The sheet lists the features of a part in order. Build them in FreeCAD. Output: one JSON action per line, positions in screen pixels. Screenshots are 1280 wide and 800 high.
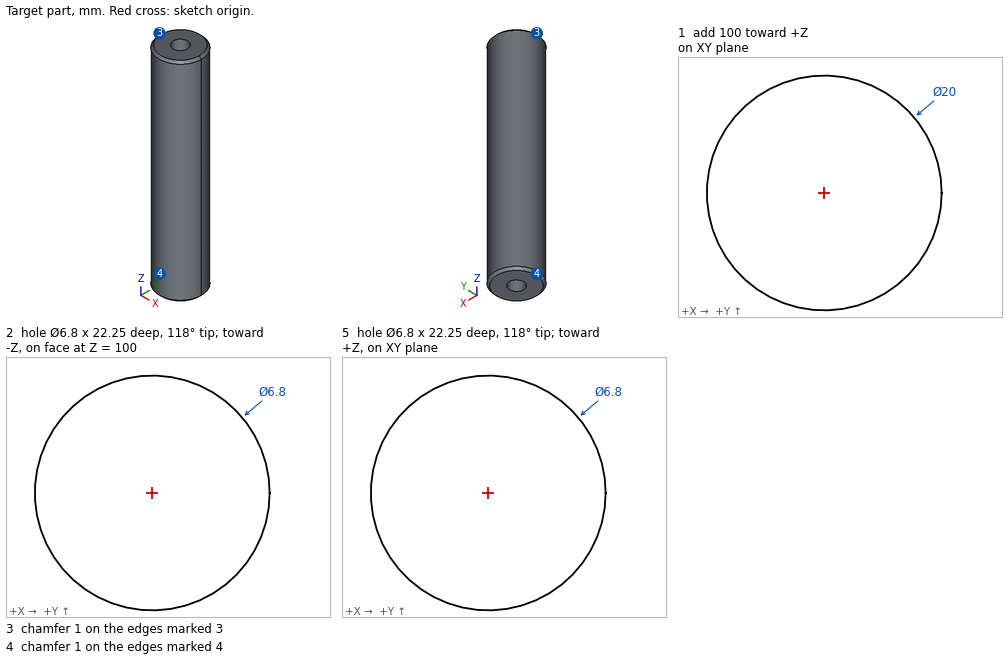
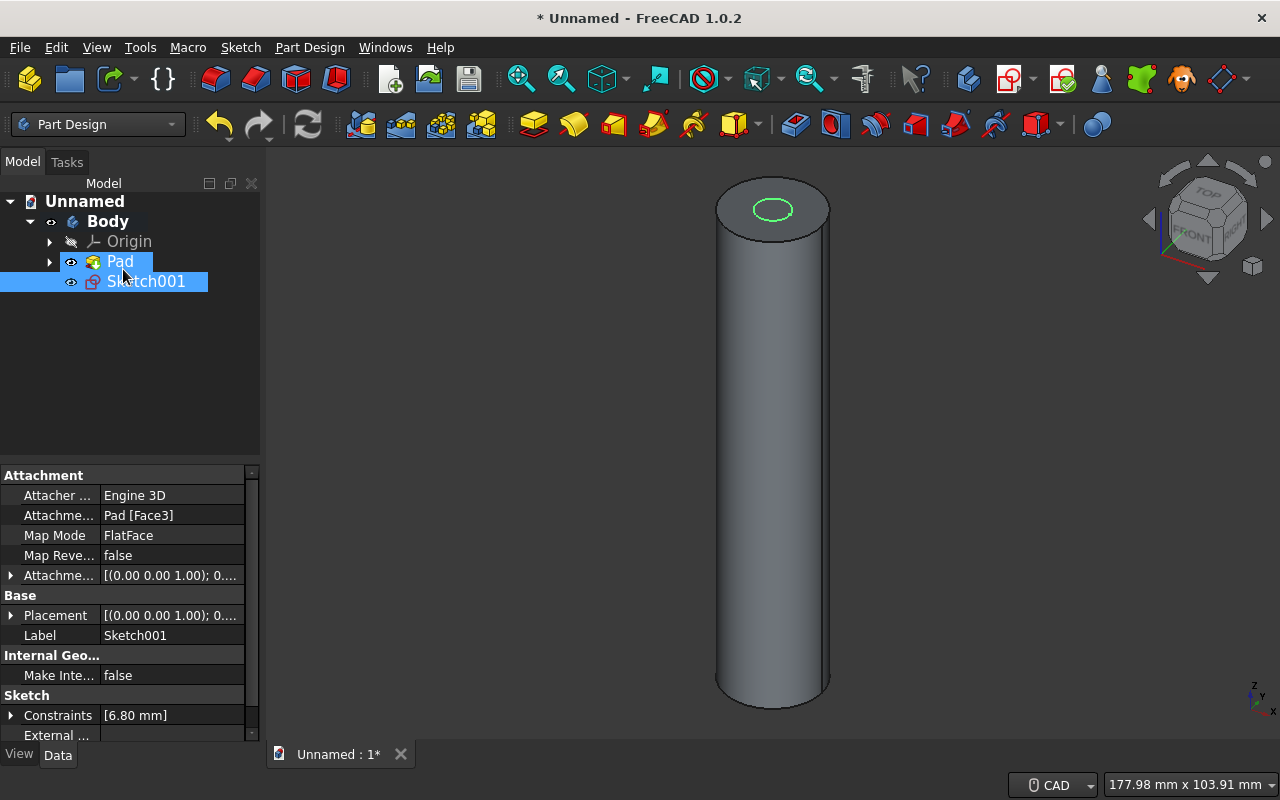
{"action": "left_click", "coordinate": [836, 124]}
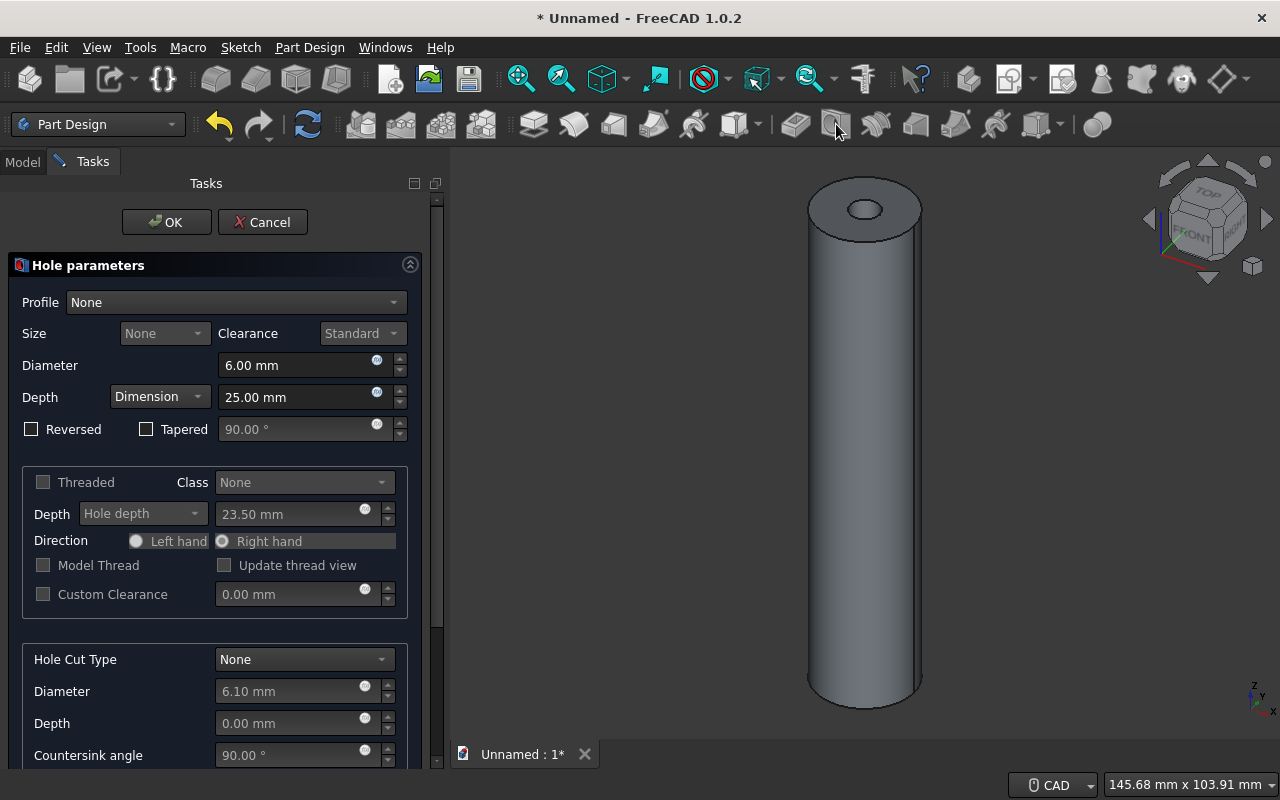
{"action": "triple_click", "coordinate": [305, 365]}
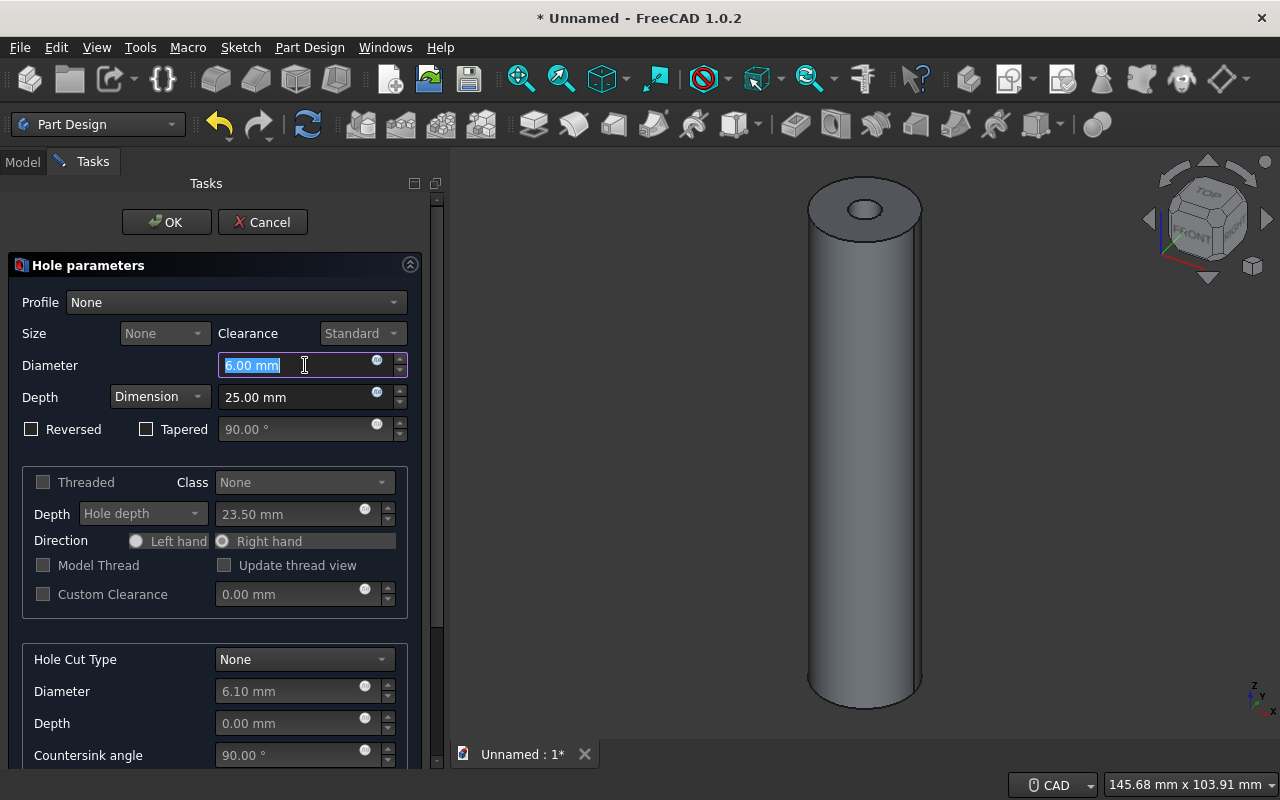
{"action": "type", "text": "6.8"}
{"action": "key", "text": "Tab"}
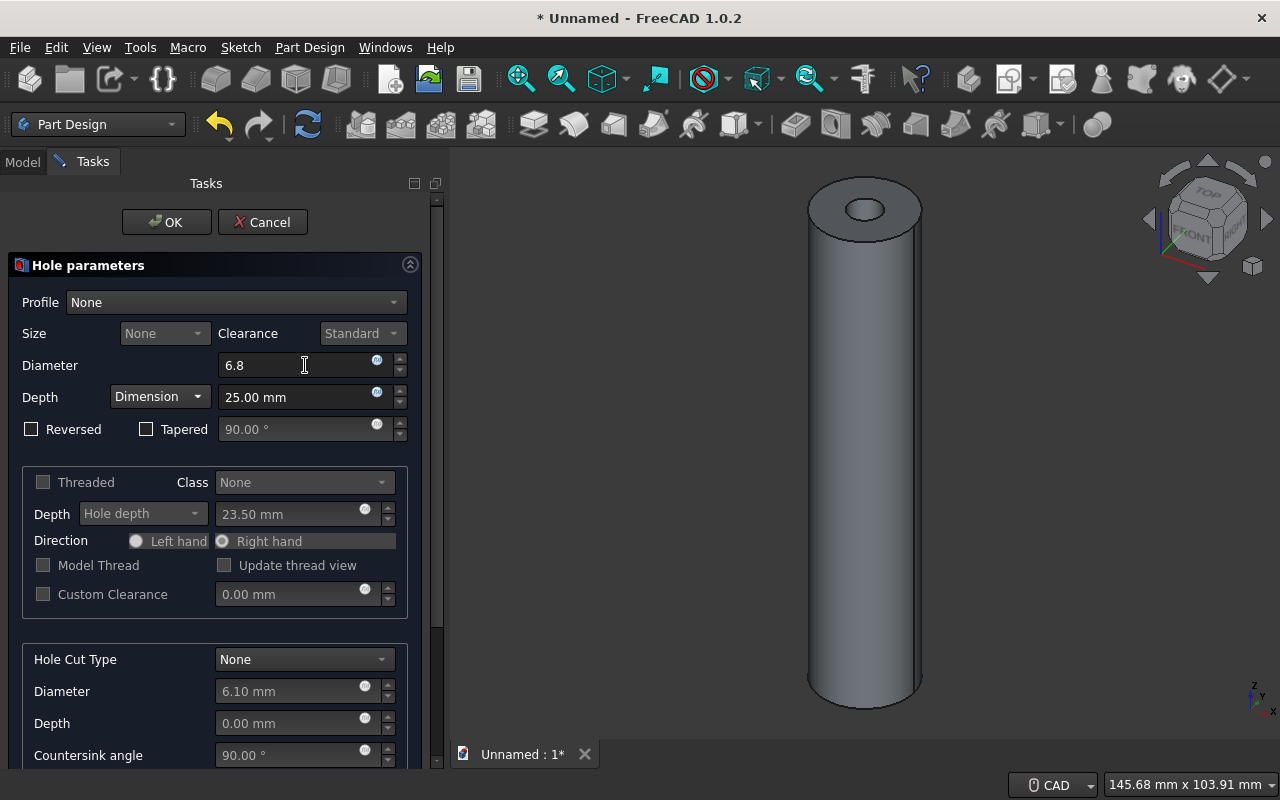
{"action": "triple_click", "coordinate": [305, 397]}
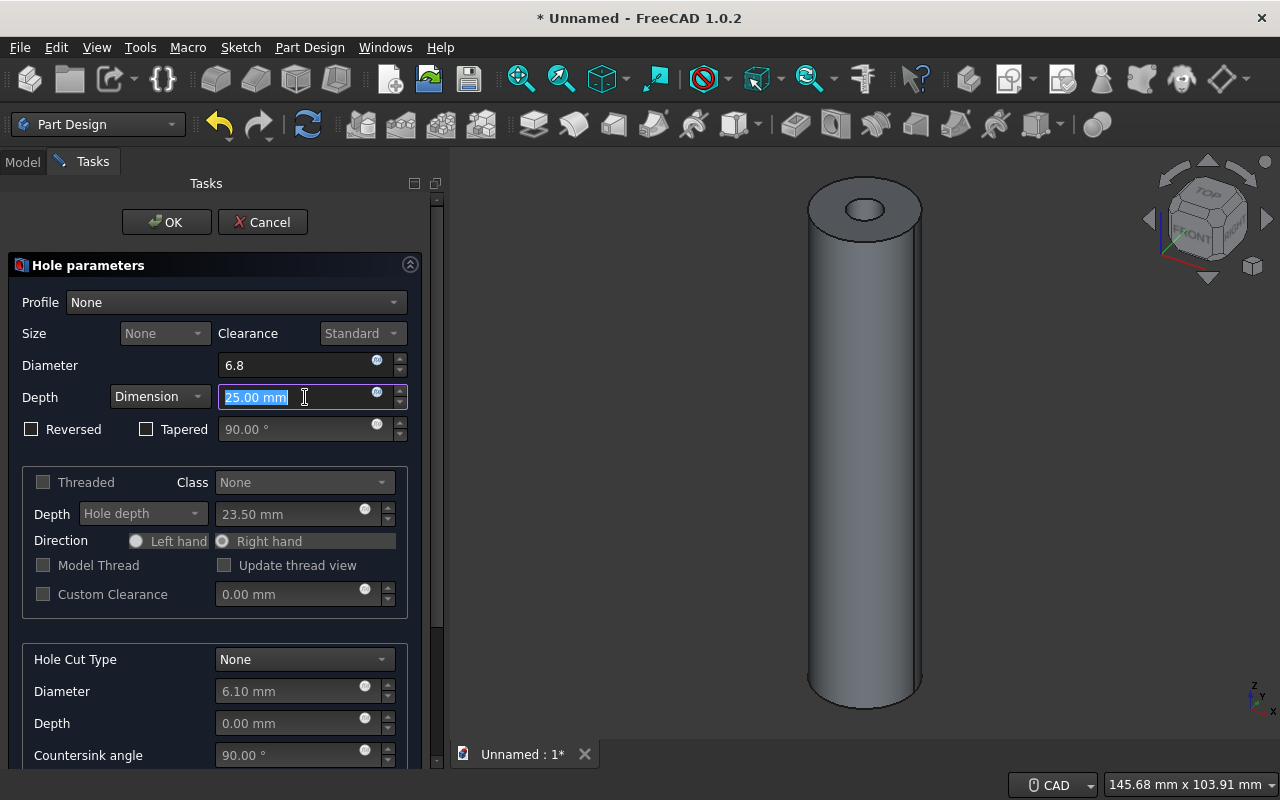
{"action": "type", "text": "22.25"}
{"action": "key", "text": "Tab"}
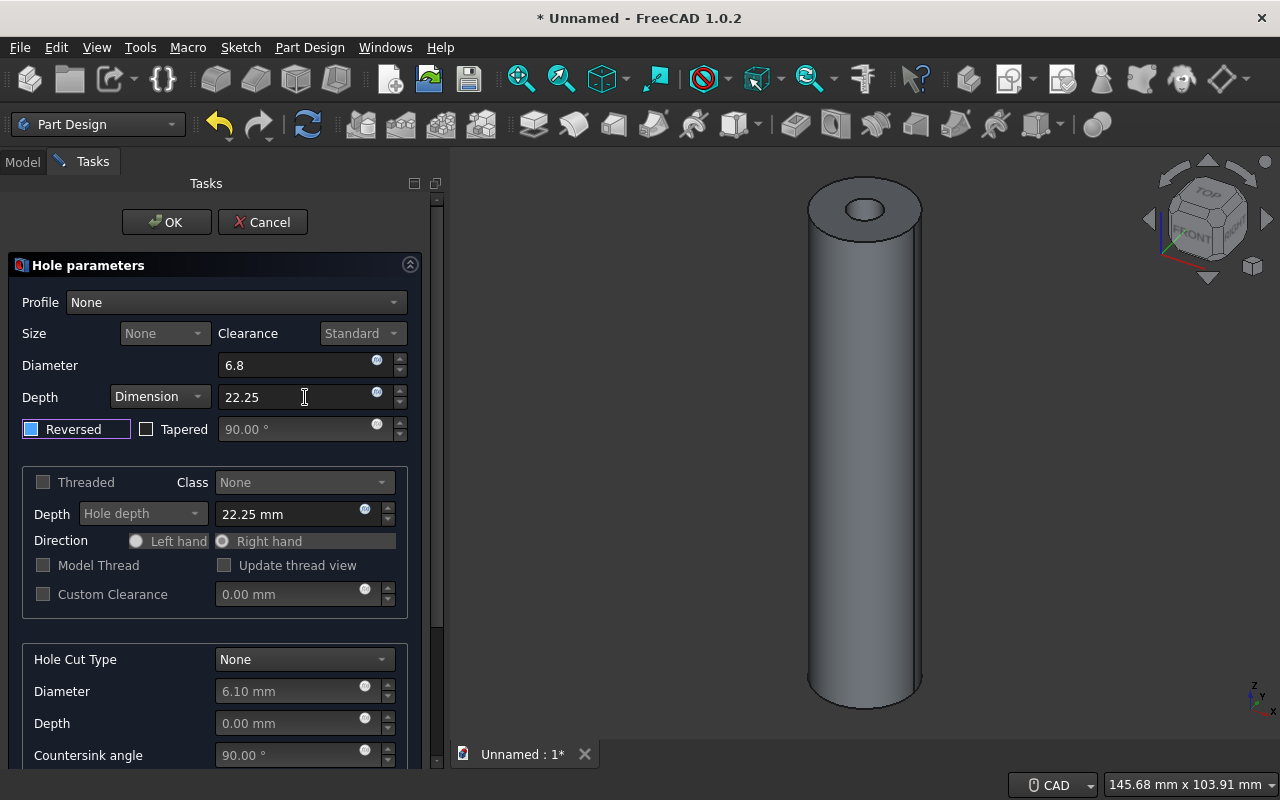
{"action": "left_click", "coordinate": [167, 222]}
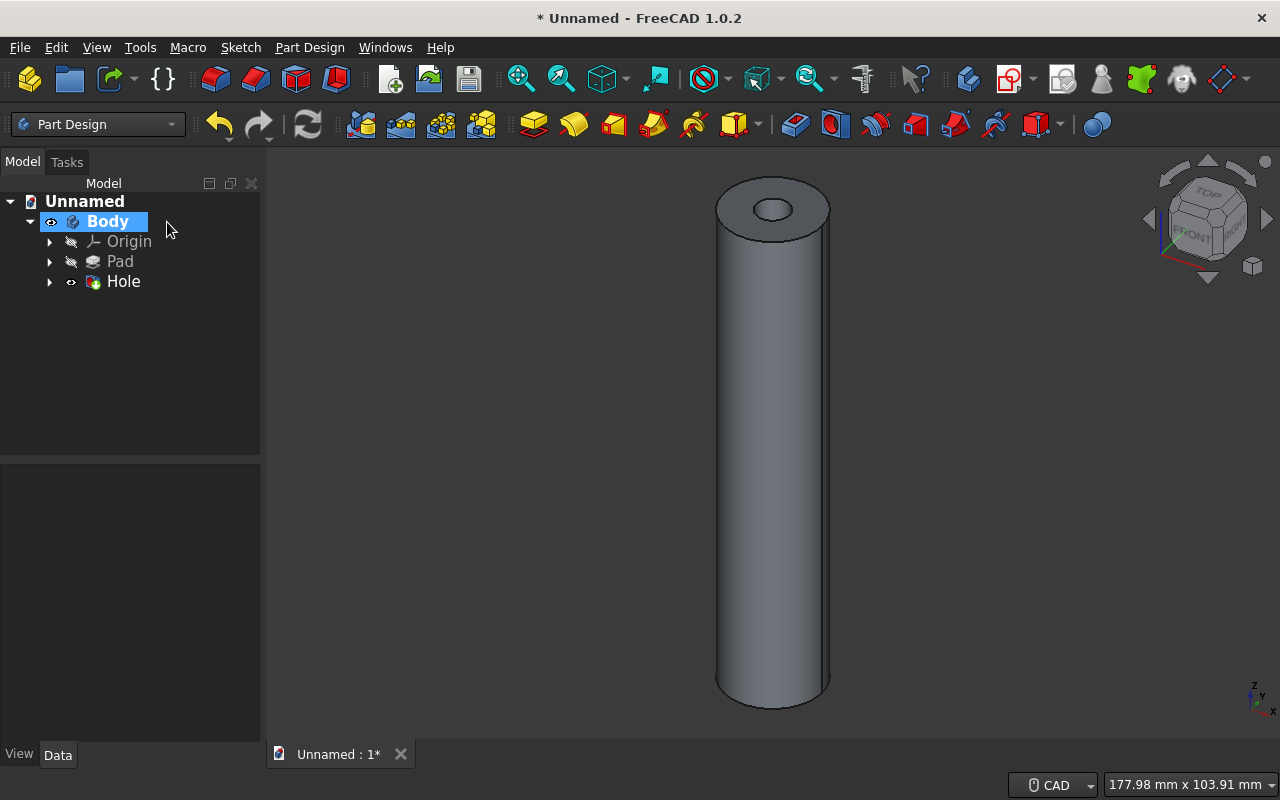
{"action": "left_click", "coordinate": [716, 212]}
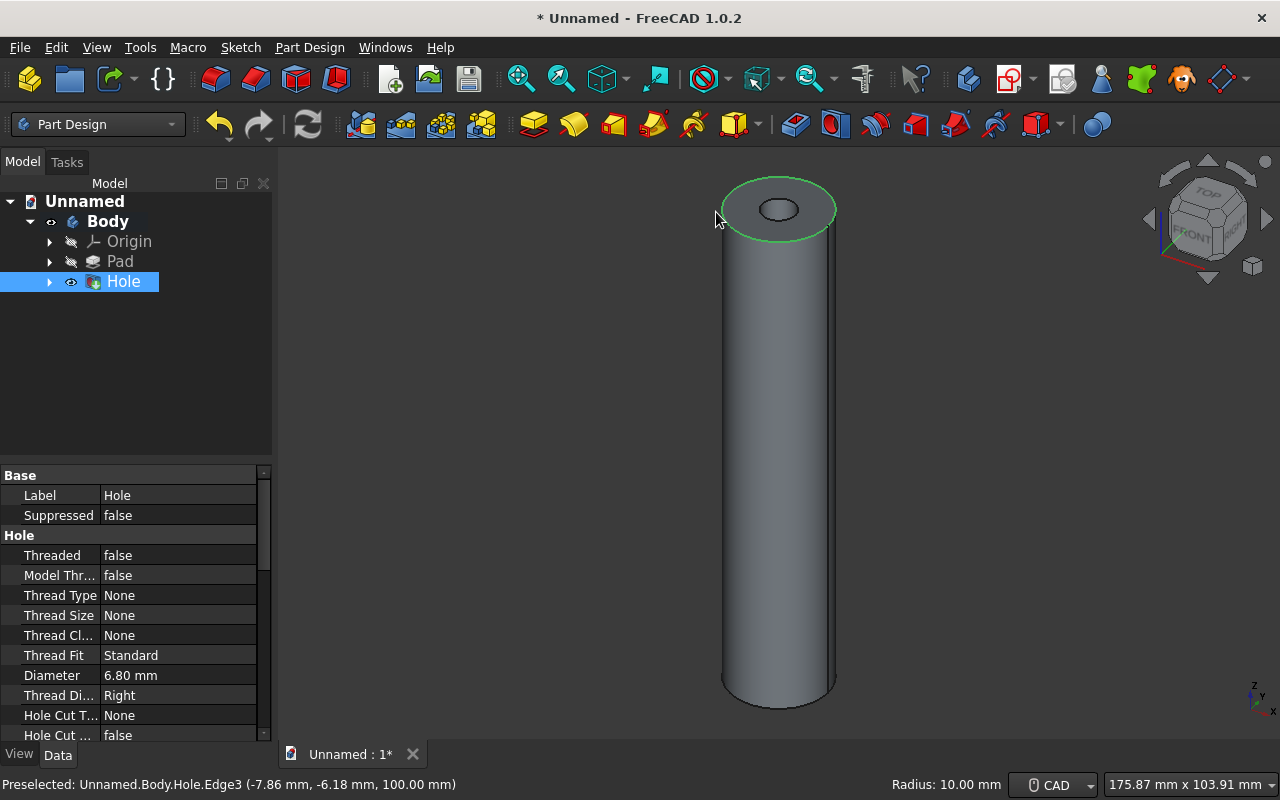
{"action": "left_click", "coordinate": [256, 80]}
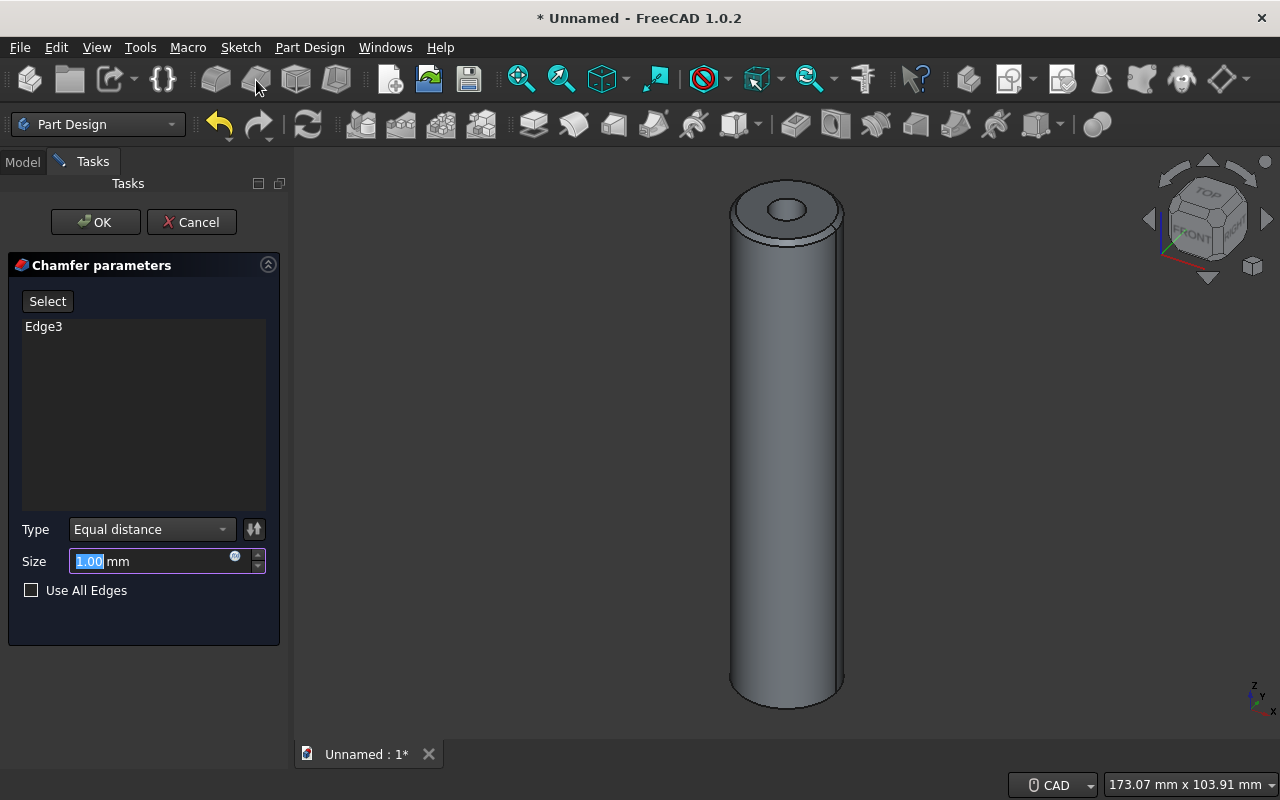
{"action": "type", "text": "1"}
{"action": "key", "text": "Tab"}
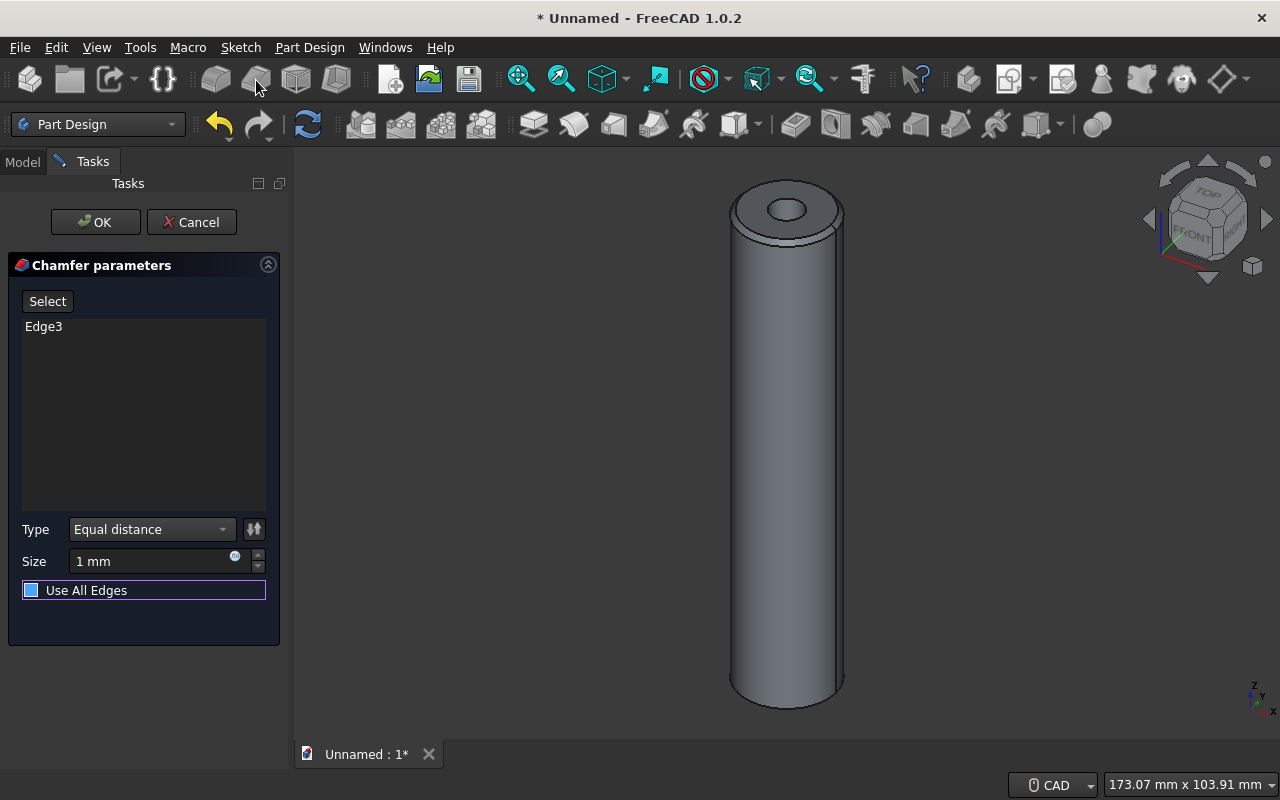
{"action": "left_click", "coordinate": [96, 222]}